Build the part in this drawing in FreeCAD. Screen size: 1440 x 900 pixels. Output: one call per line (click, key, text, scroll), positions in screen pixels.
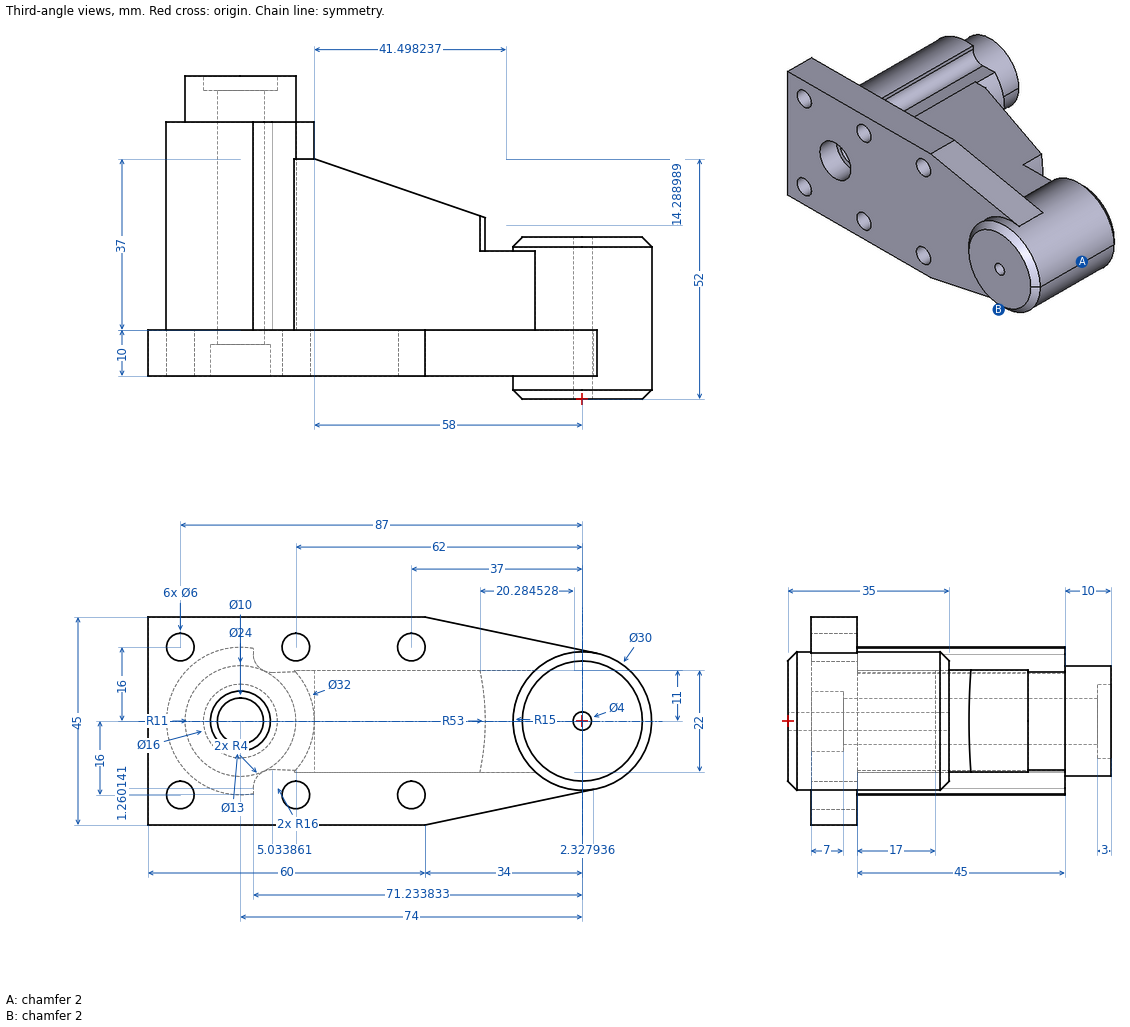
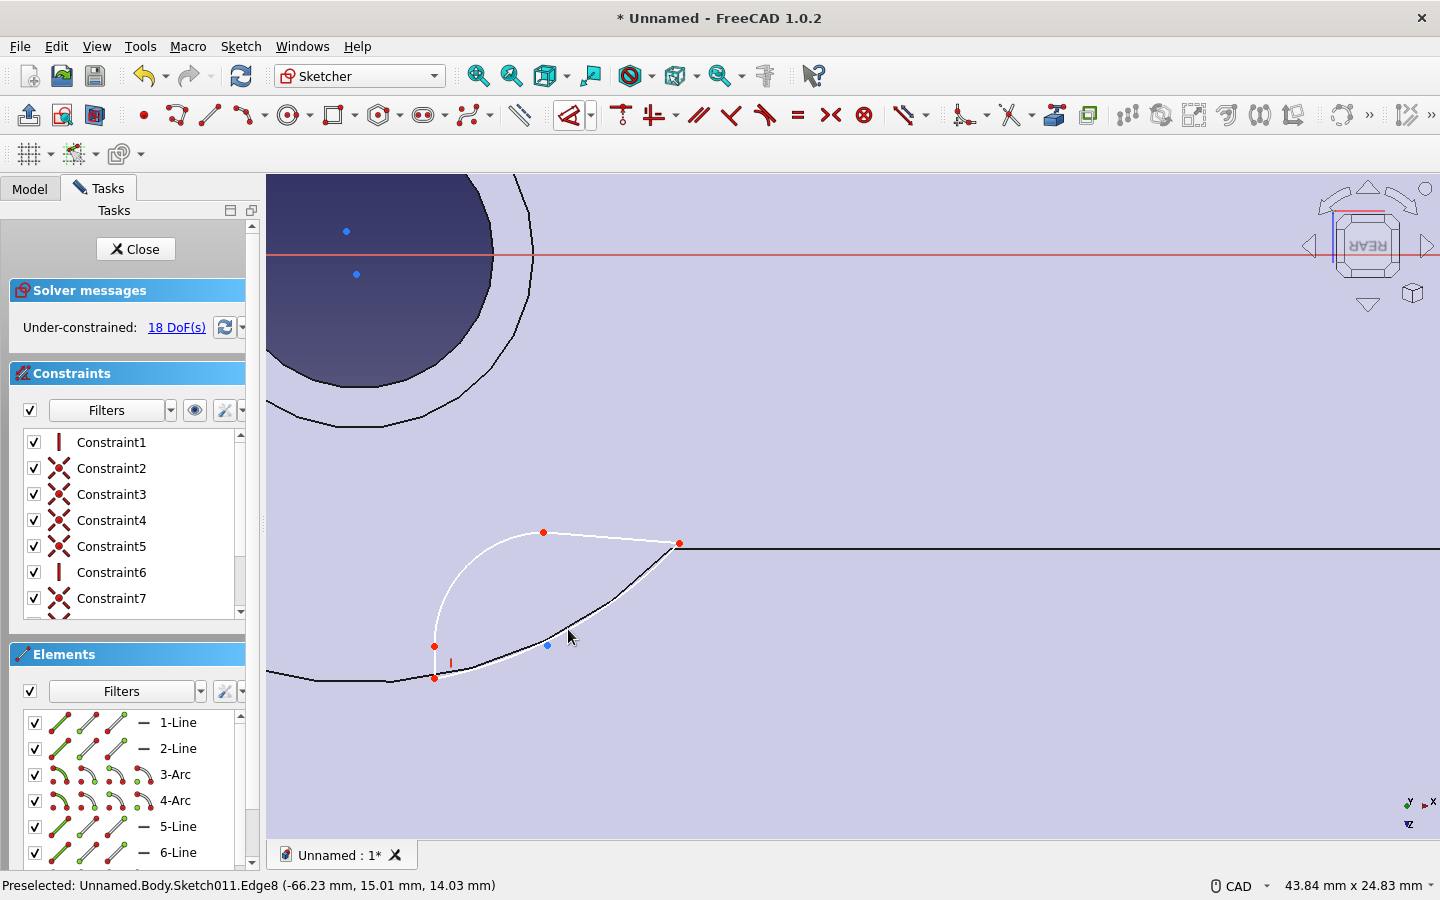
scroll(434, 653, down, 5)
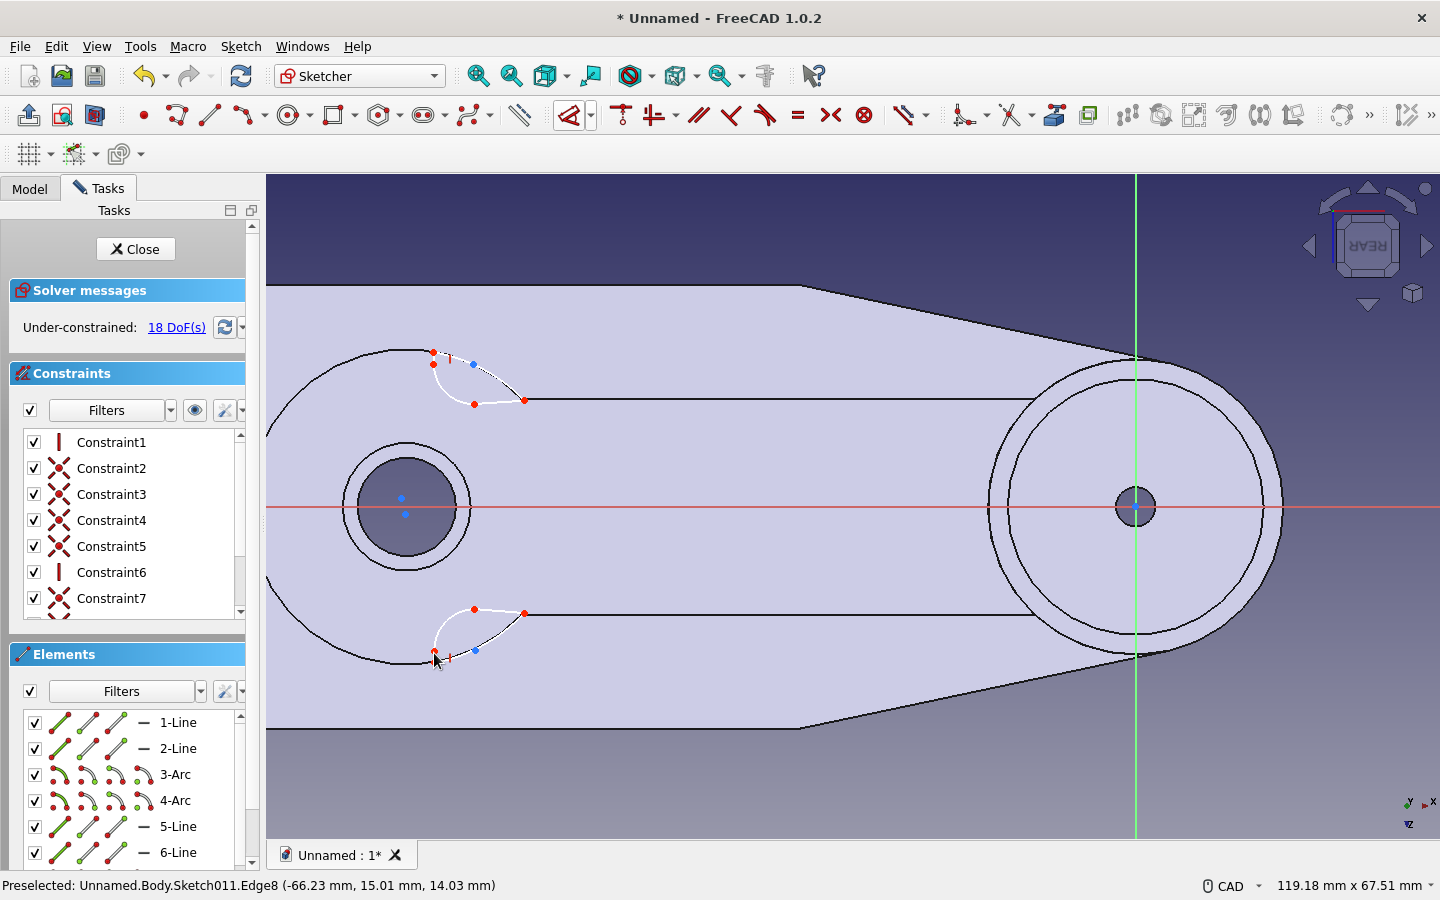
scroll(434, 356, up, 7)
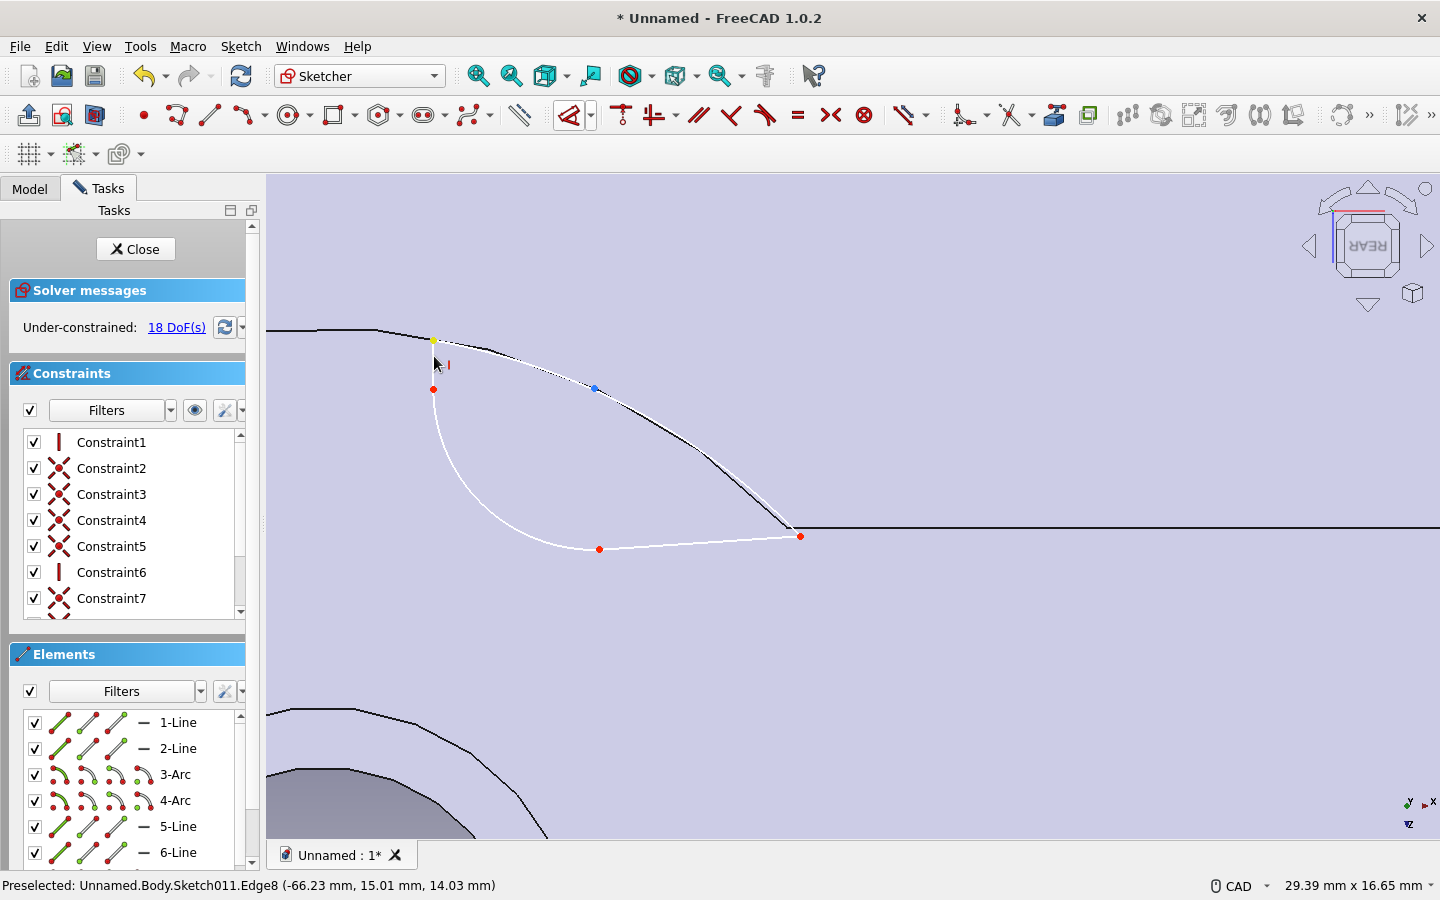
click(433, 355)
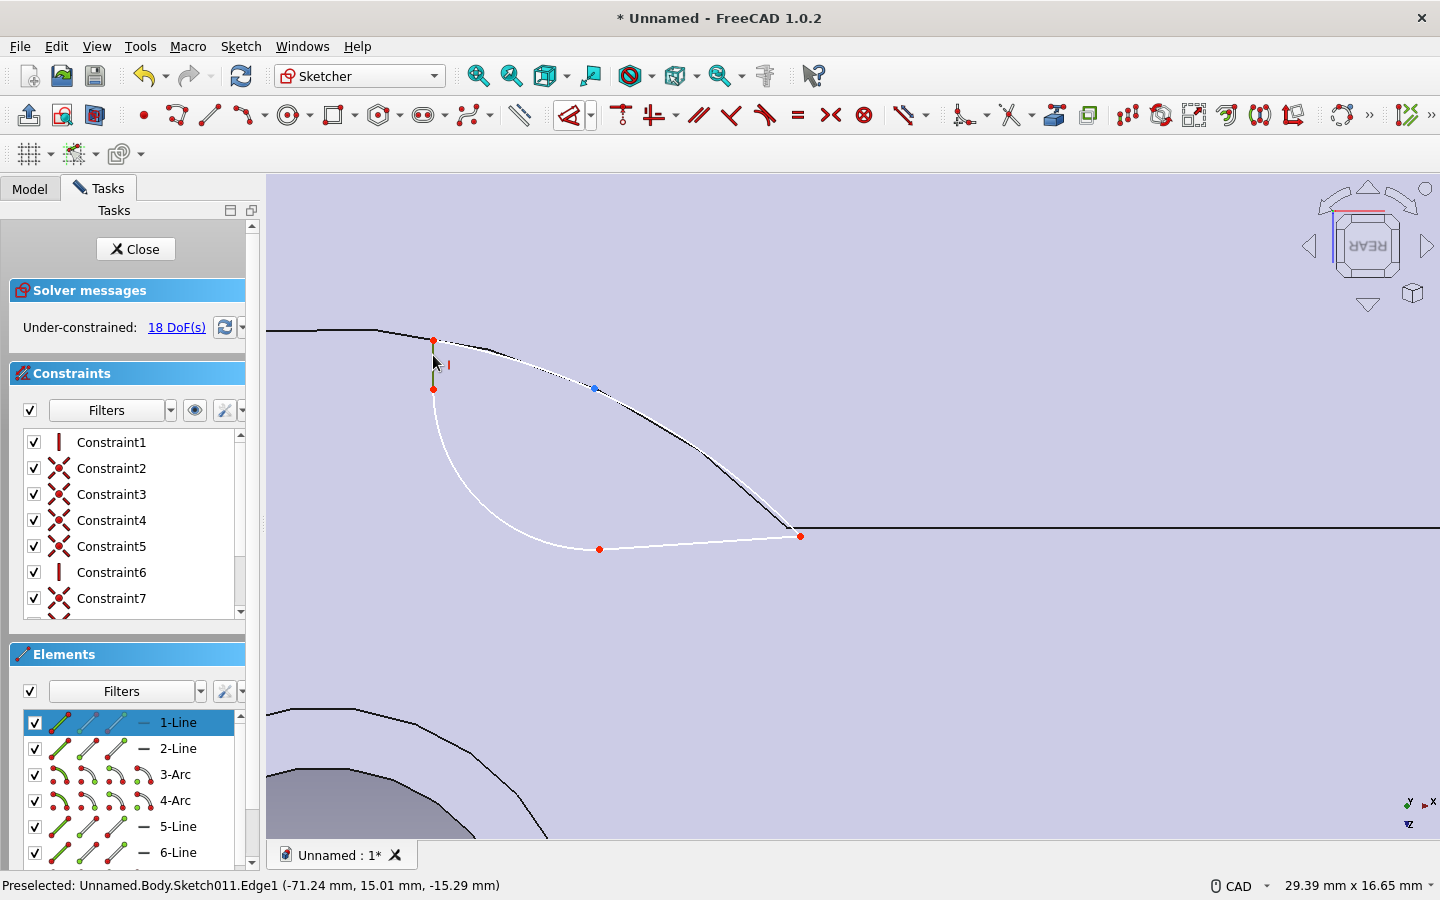
scroll(434, 356, down, 7)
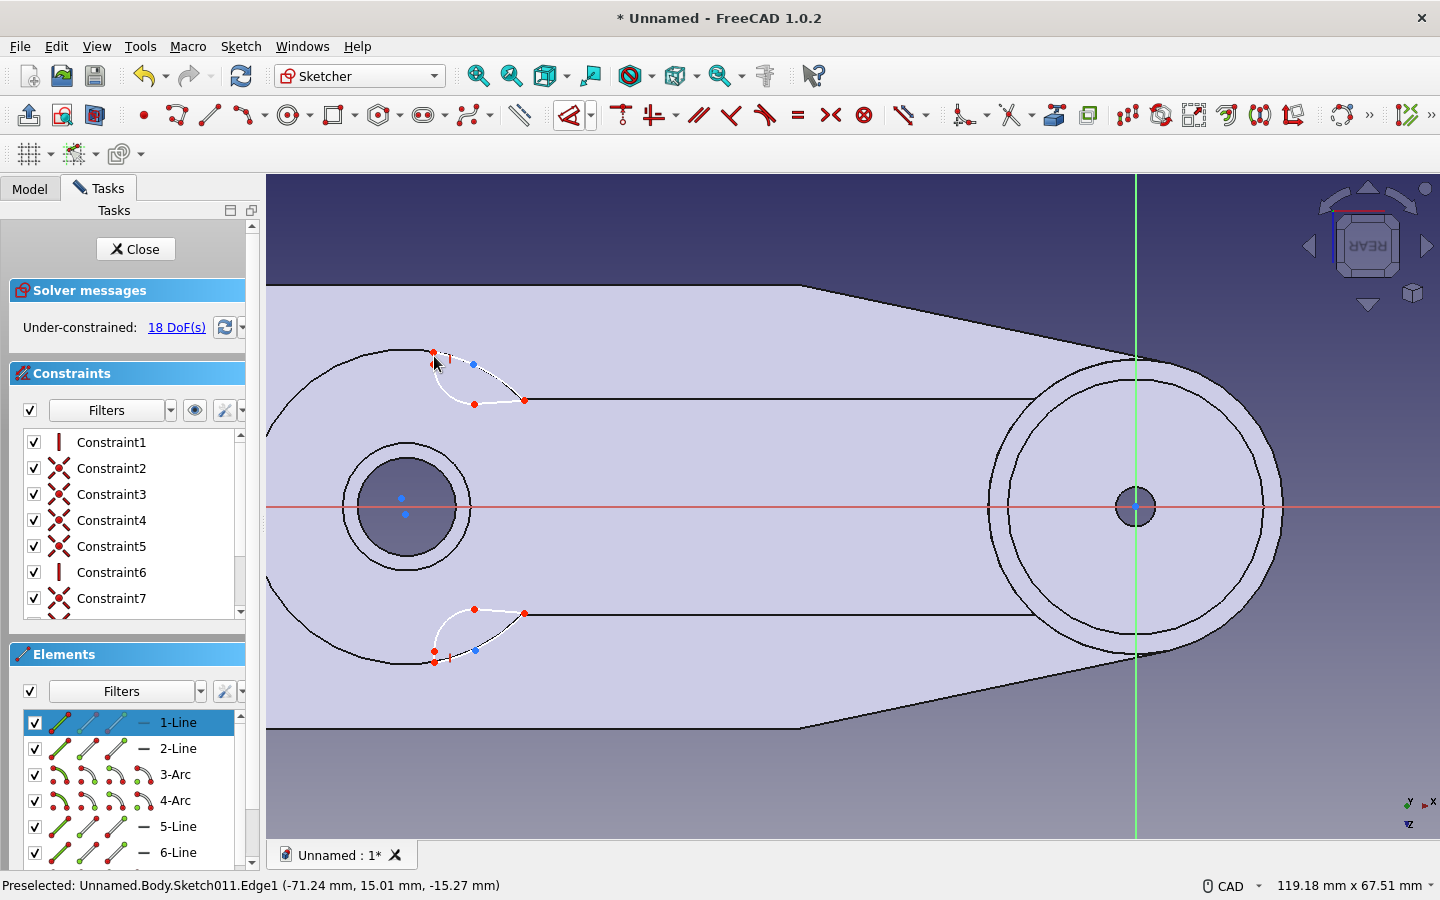
click(439, 383)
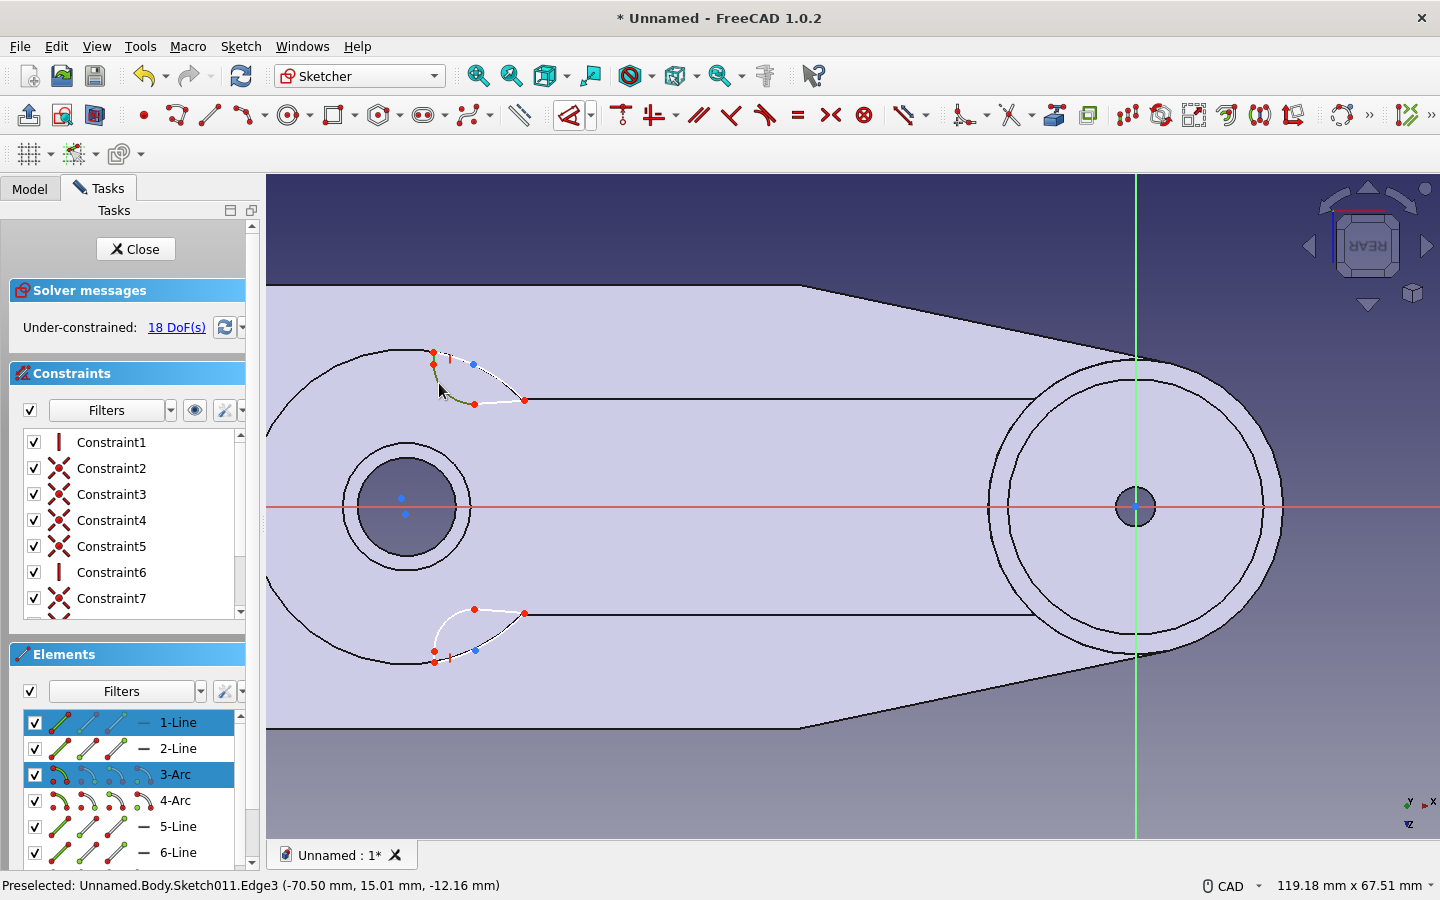
click(765, 116)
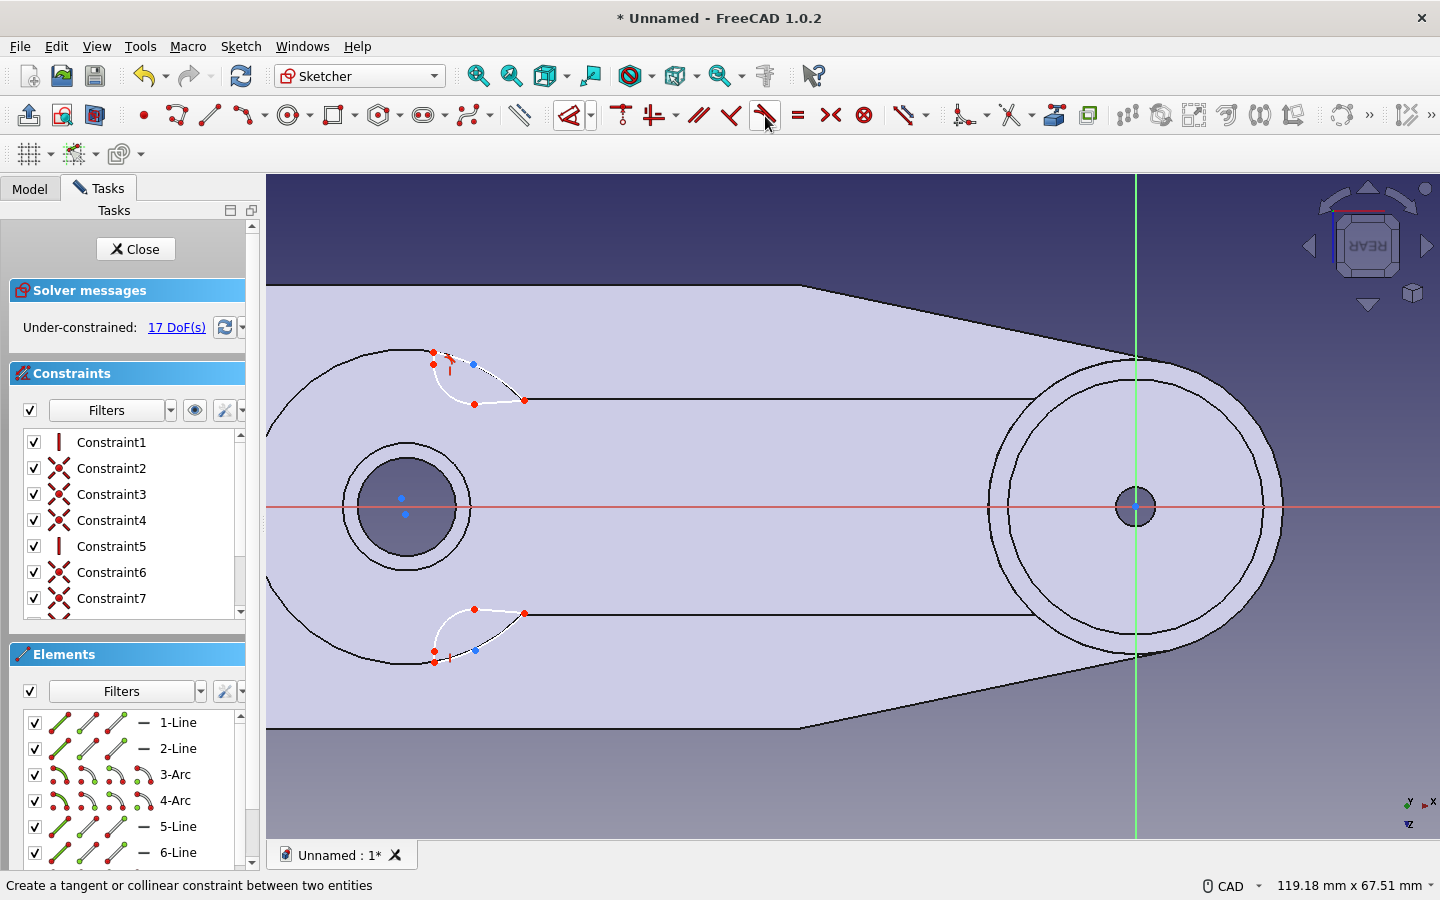
click(490, 403)